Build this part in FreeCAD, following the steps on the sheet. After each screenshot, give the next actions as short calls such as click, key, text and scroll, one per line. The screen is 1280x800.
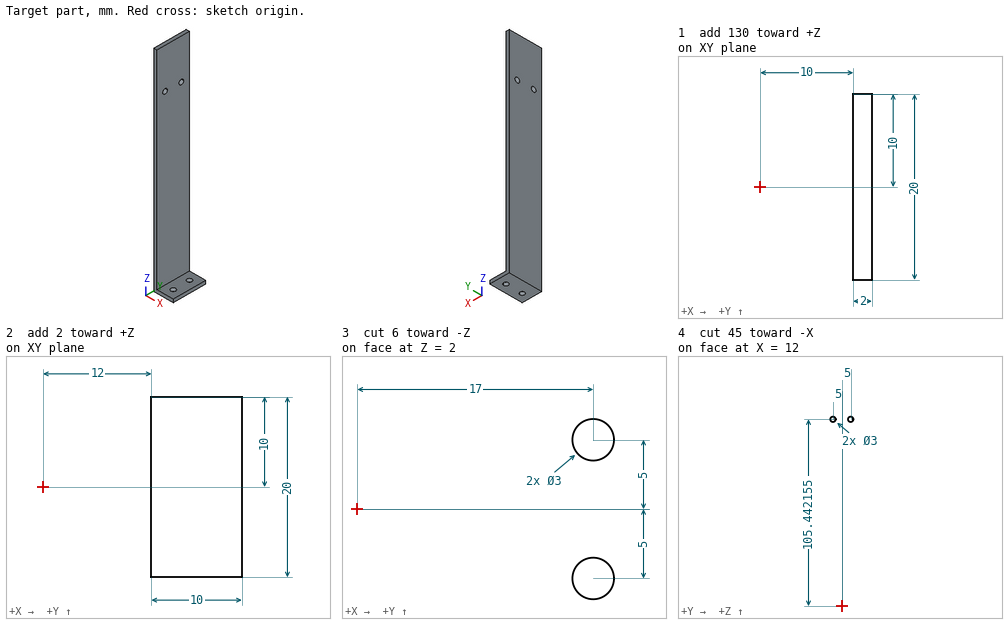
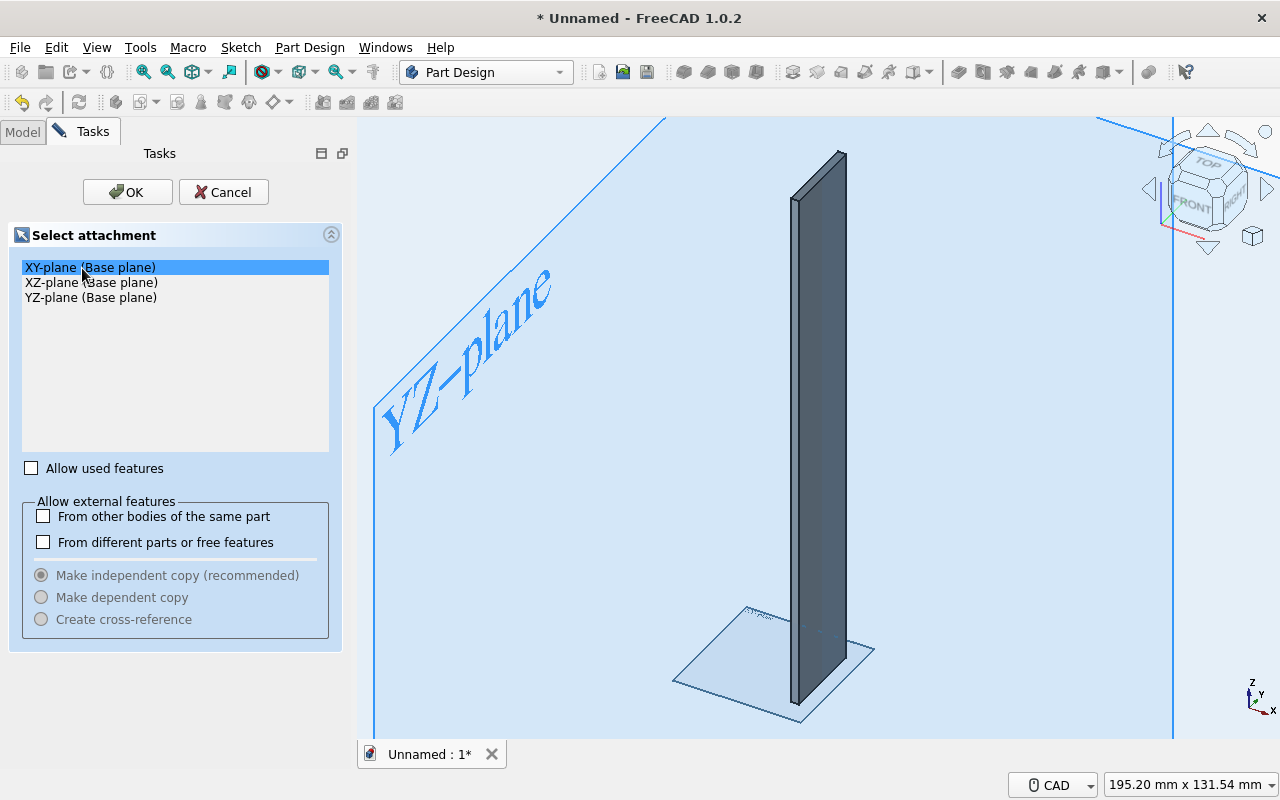
click(128, 192)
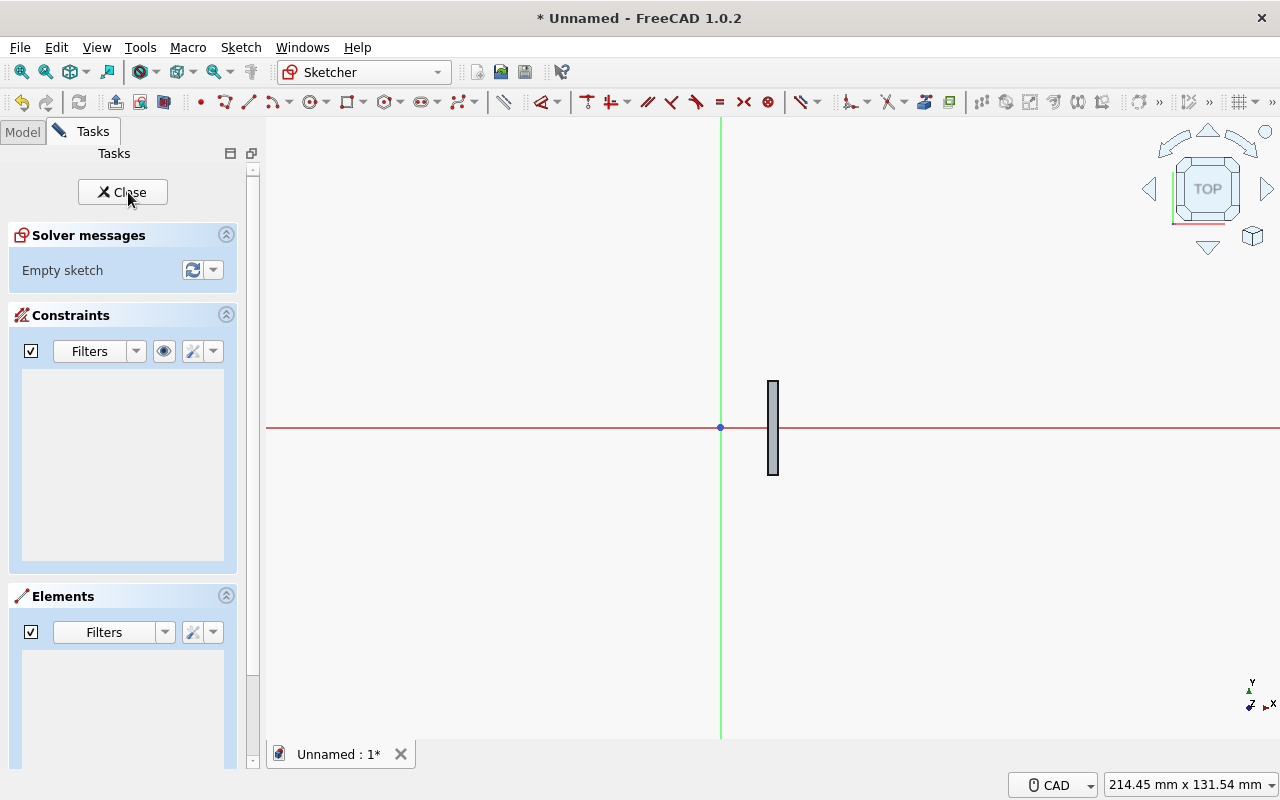
key(q)
key(s)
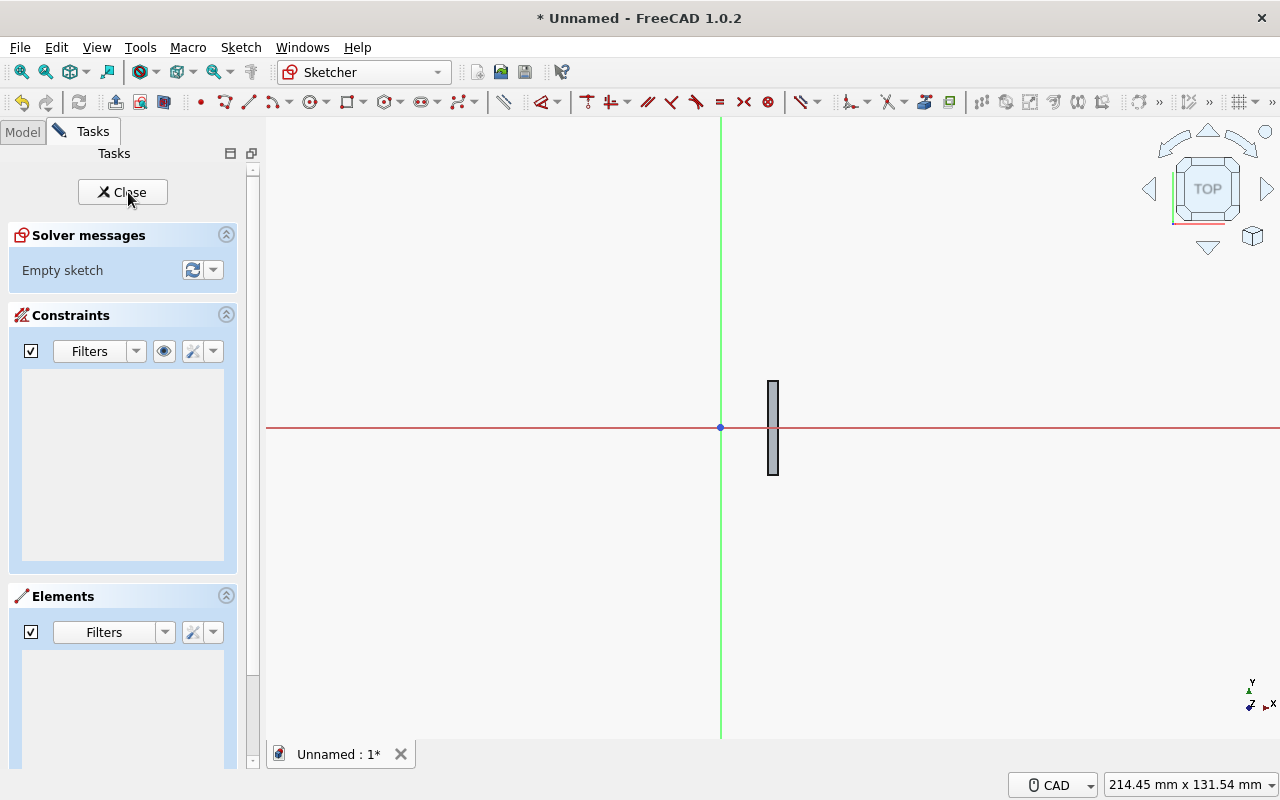
scroll(795, 428, up, 7)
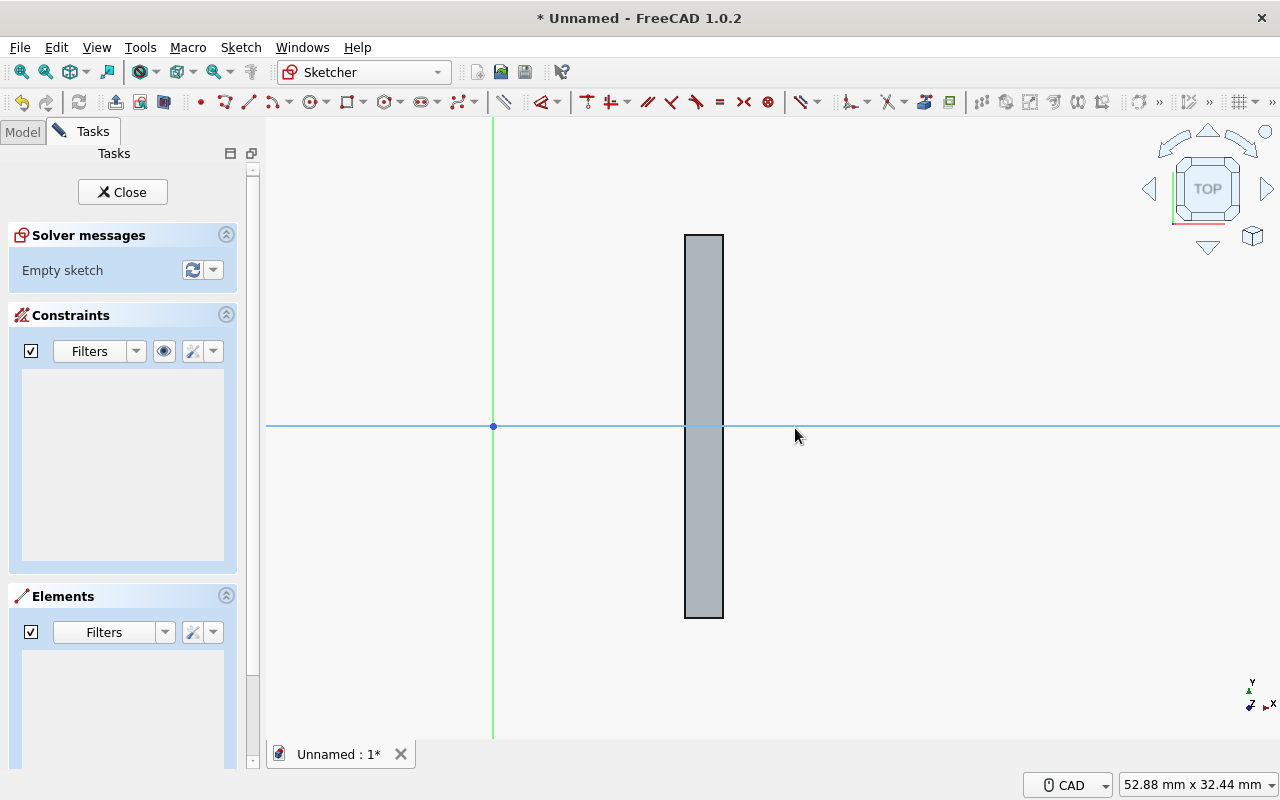
click(348, 102)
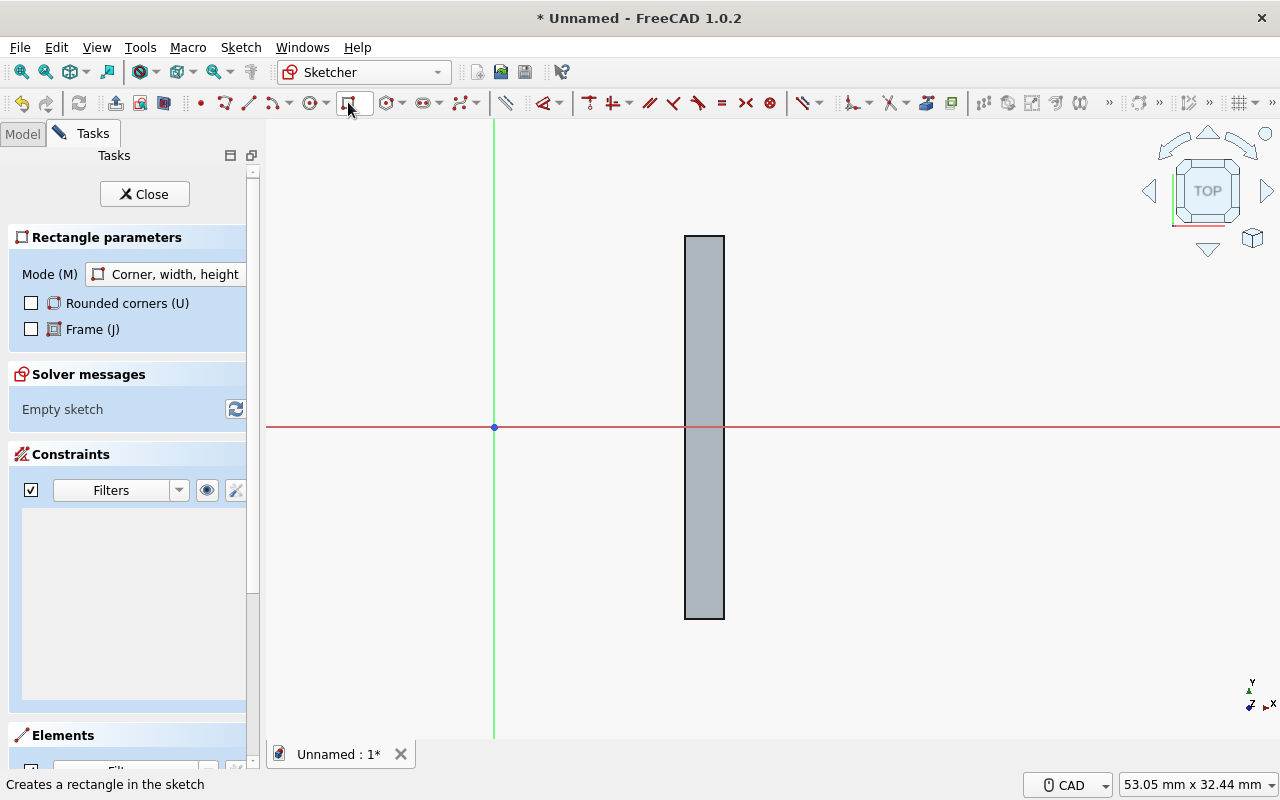
click(724, 236)
move(915, 619)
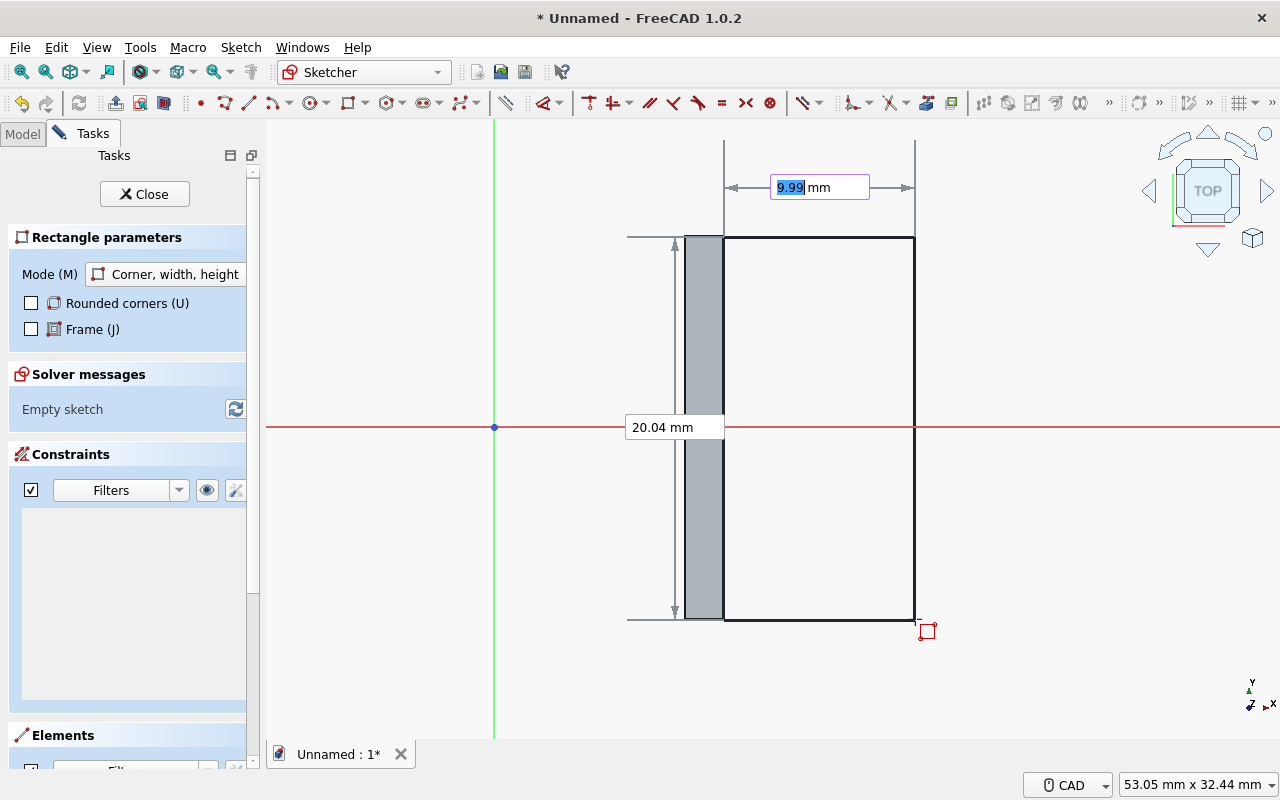
text(10)
key(Tab)
text(20)
key(Return)
key(Escape)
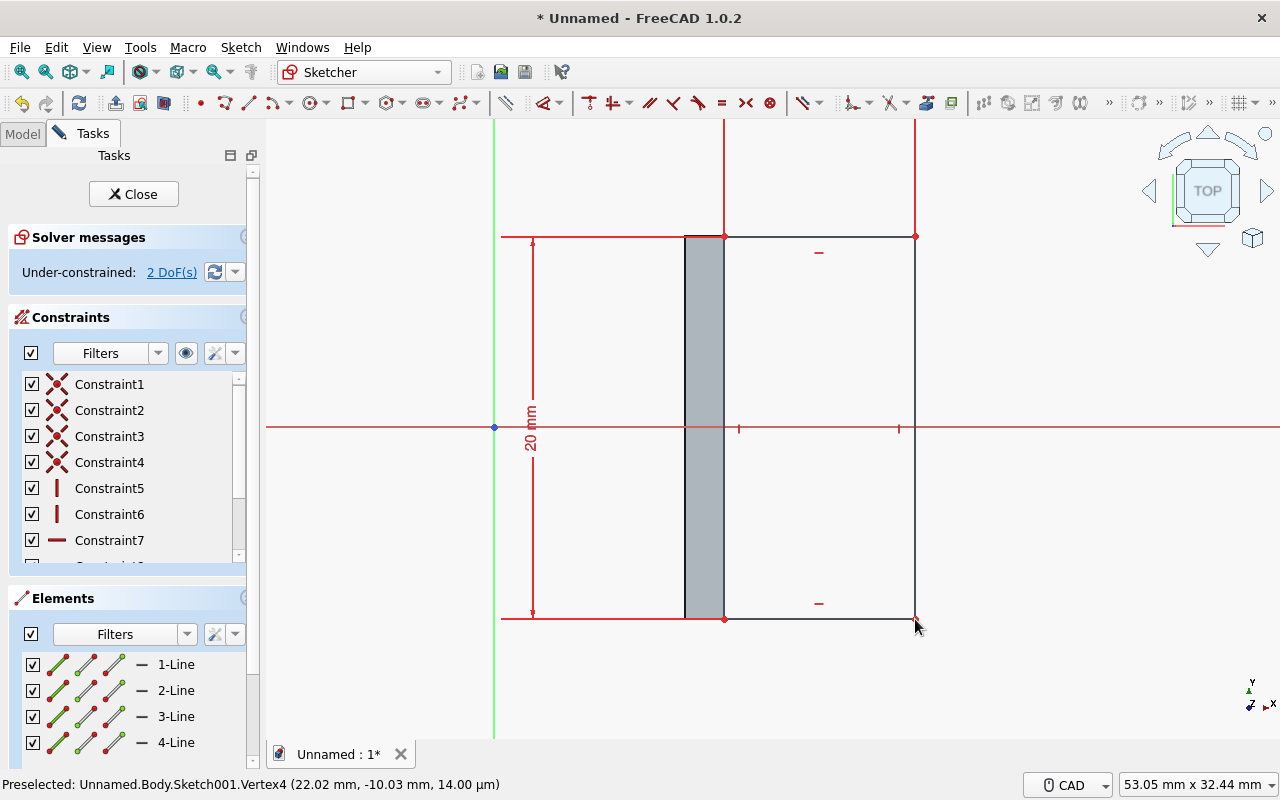
key(d)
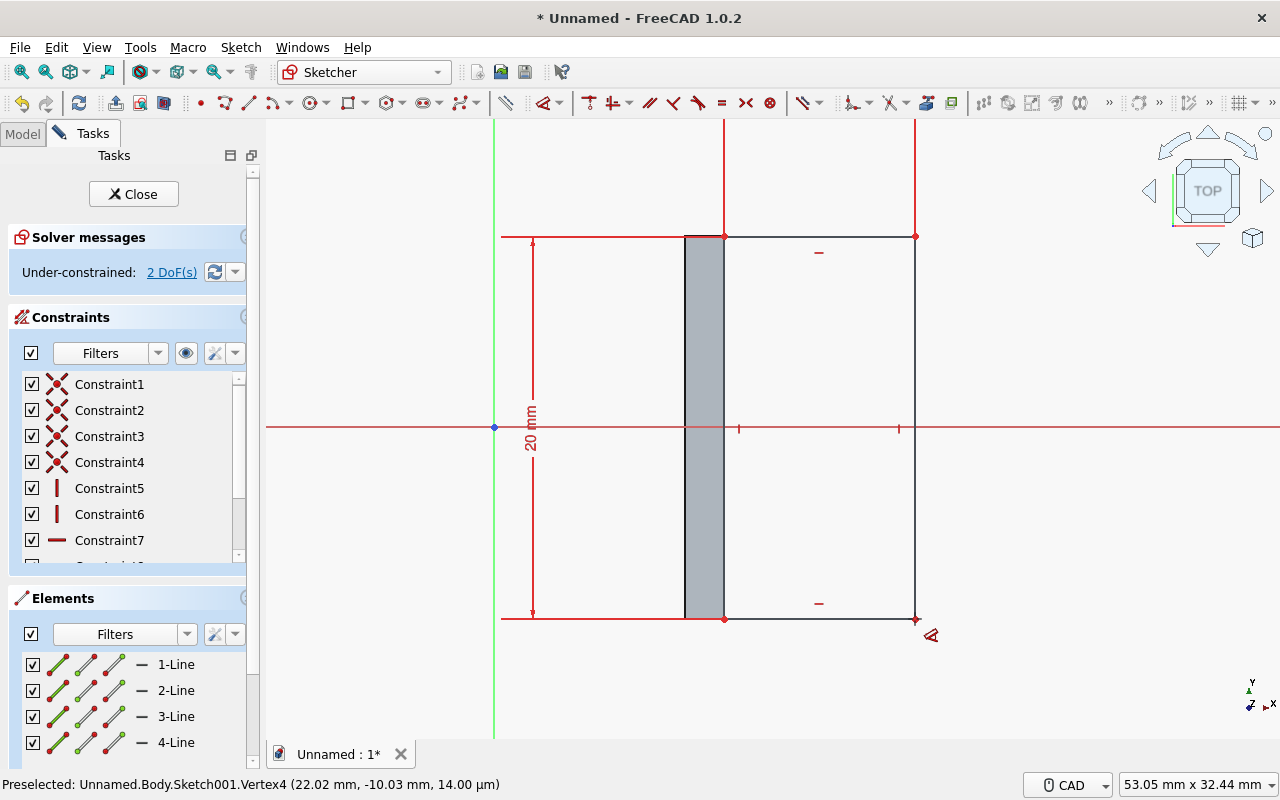
click(724, 237)
click(609, 203)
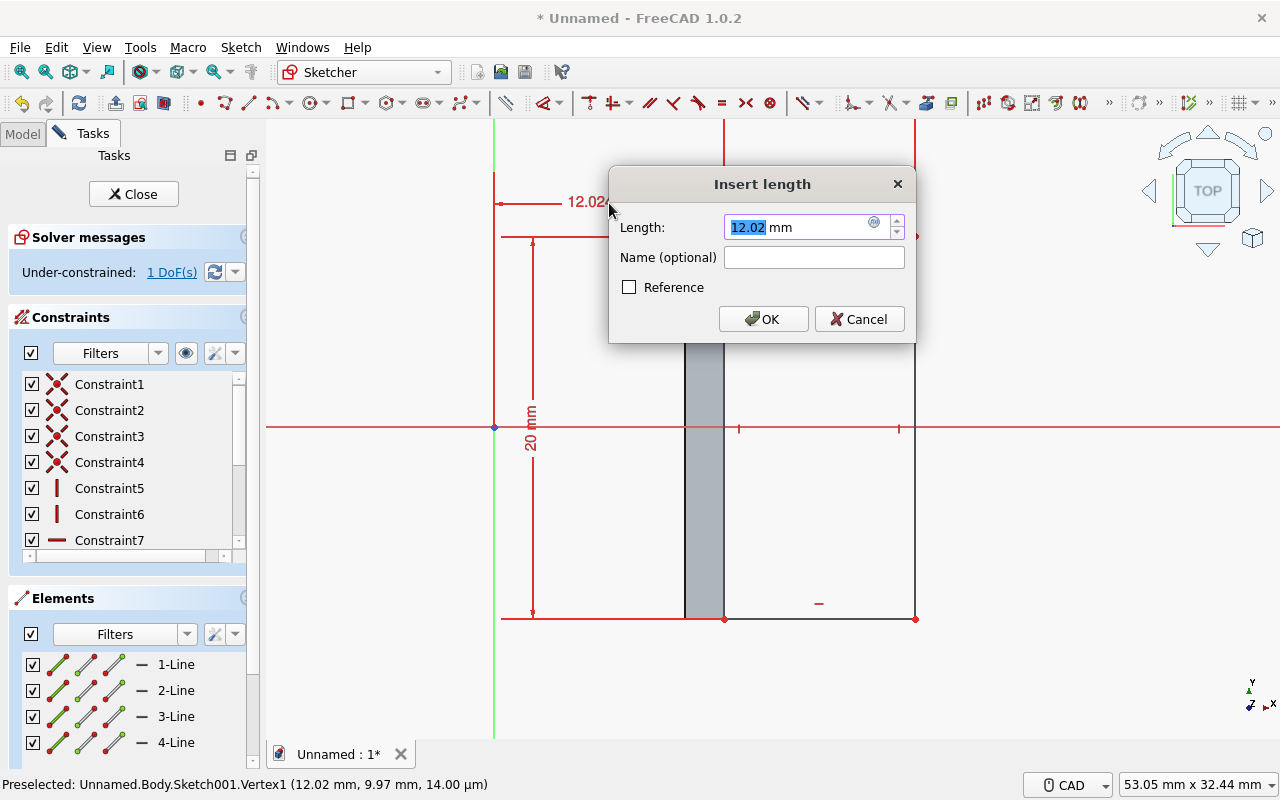
text(12)
key(Return)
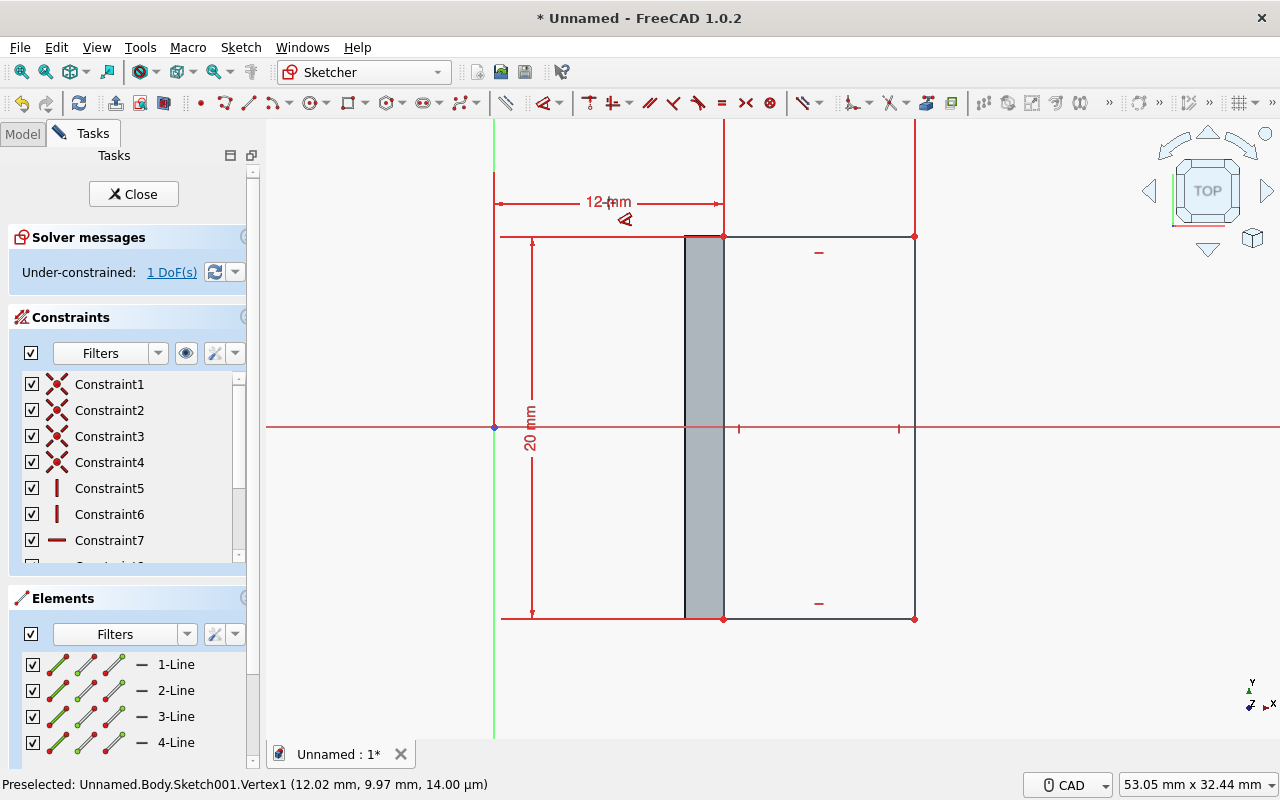
click(724, 237)
click(460, 332)